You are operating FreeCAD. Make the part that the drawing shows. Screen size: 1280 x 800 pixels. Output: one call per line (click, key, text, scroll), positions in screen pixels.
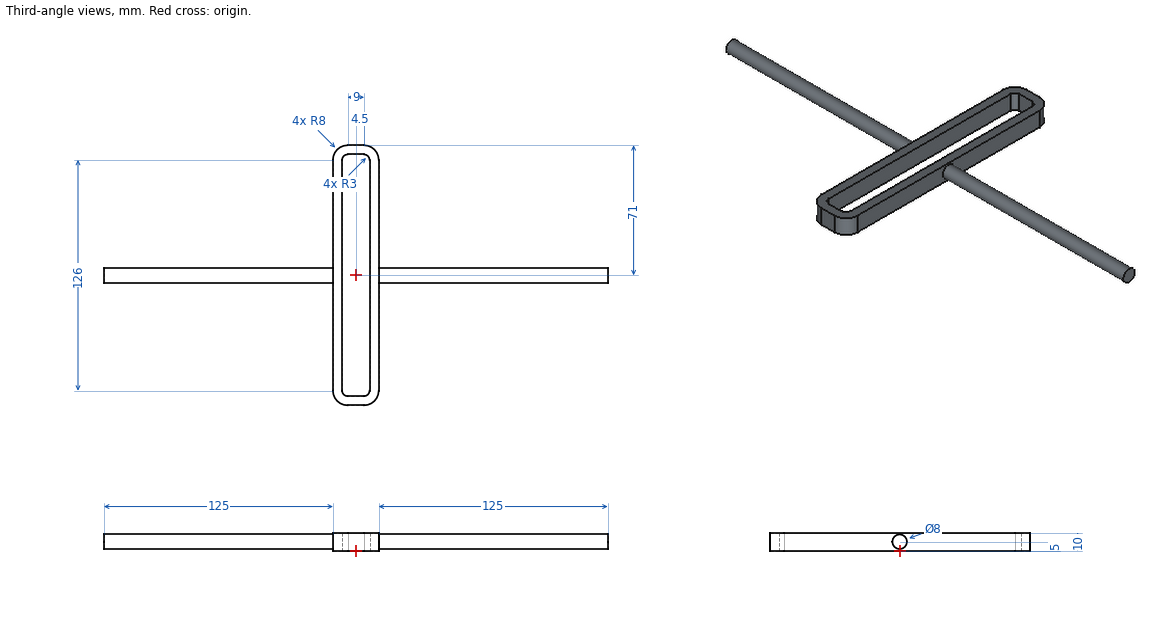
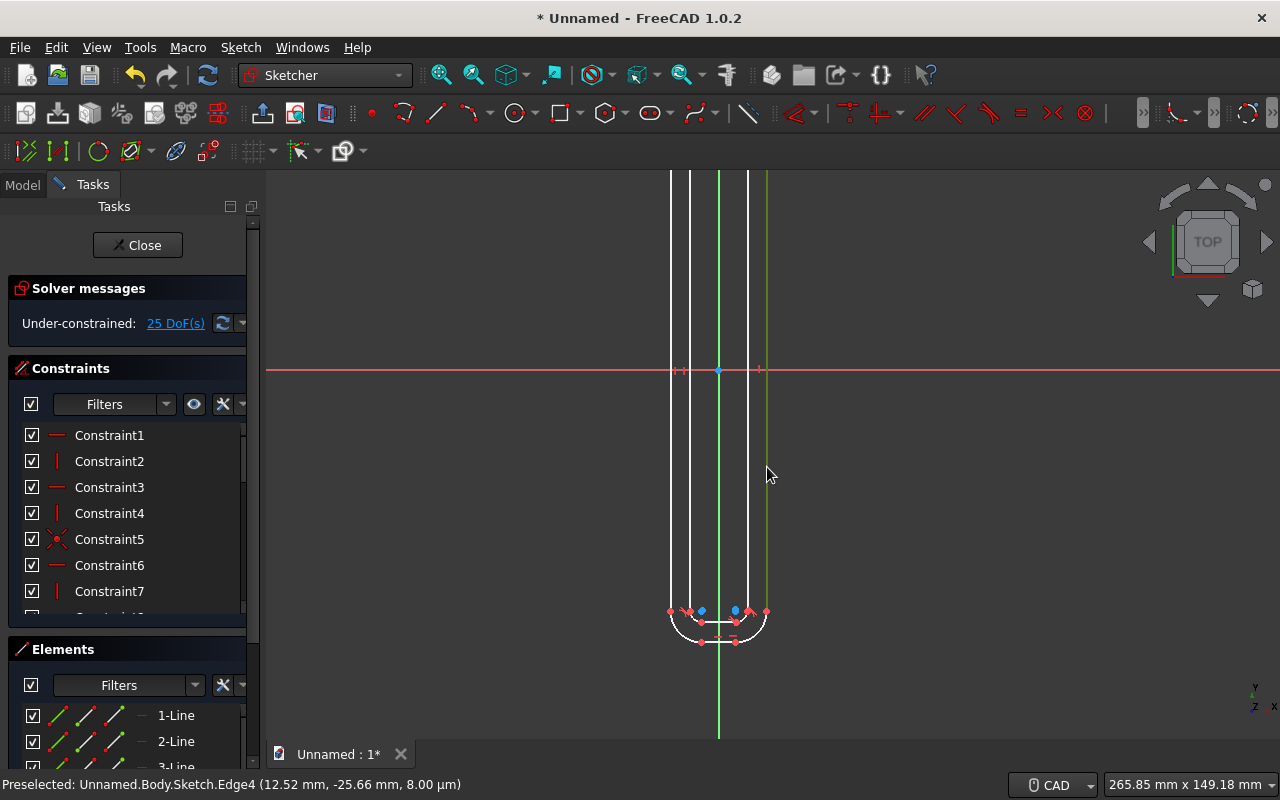
scroll(675, 626, down, 2)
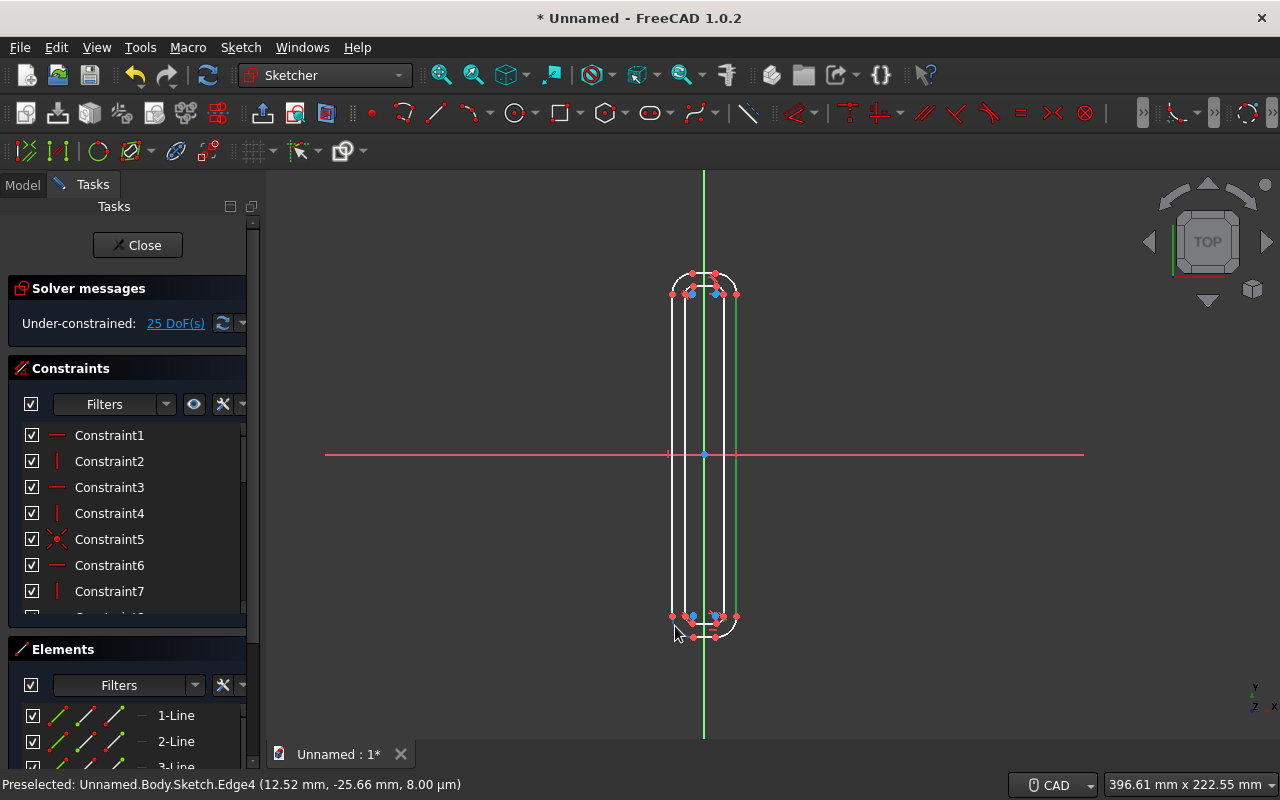
scroll(734, 285, up, 2)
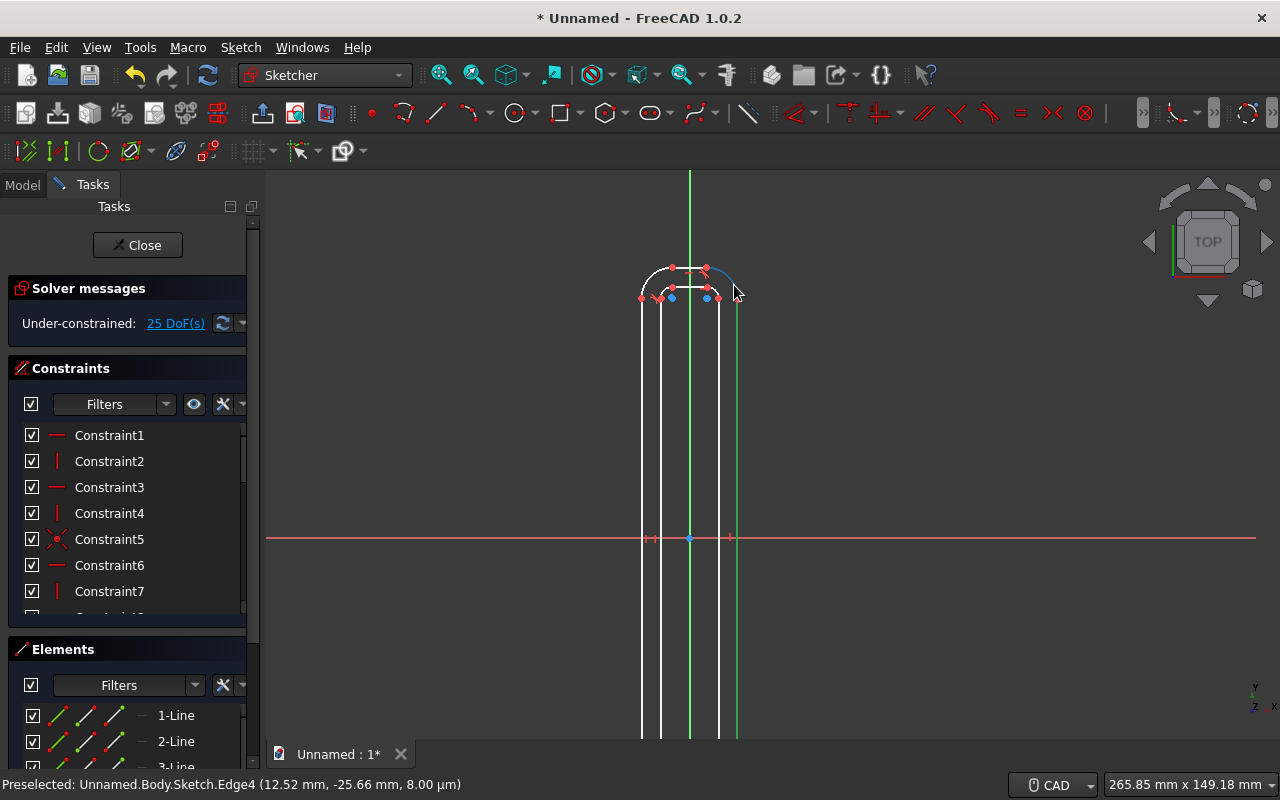
click(734, 285)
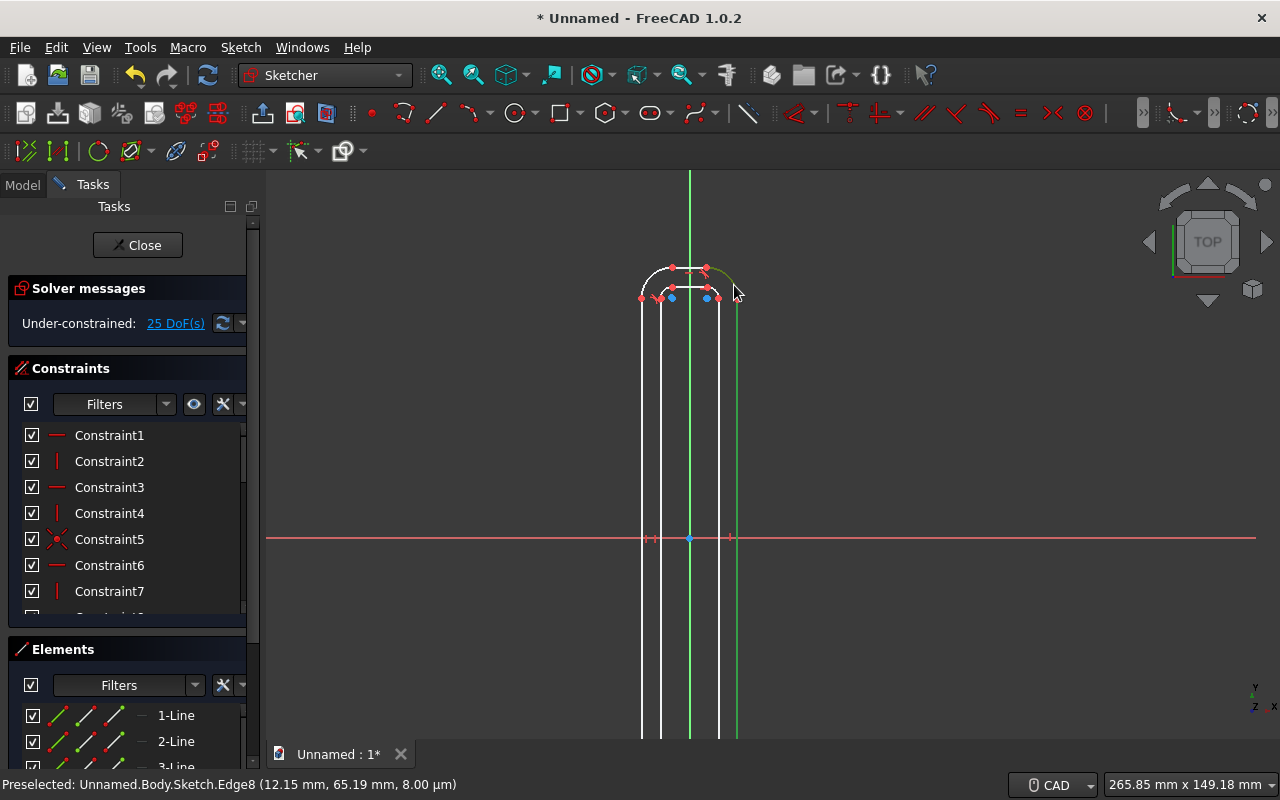
click(990, 114)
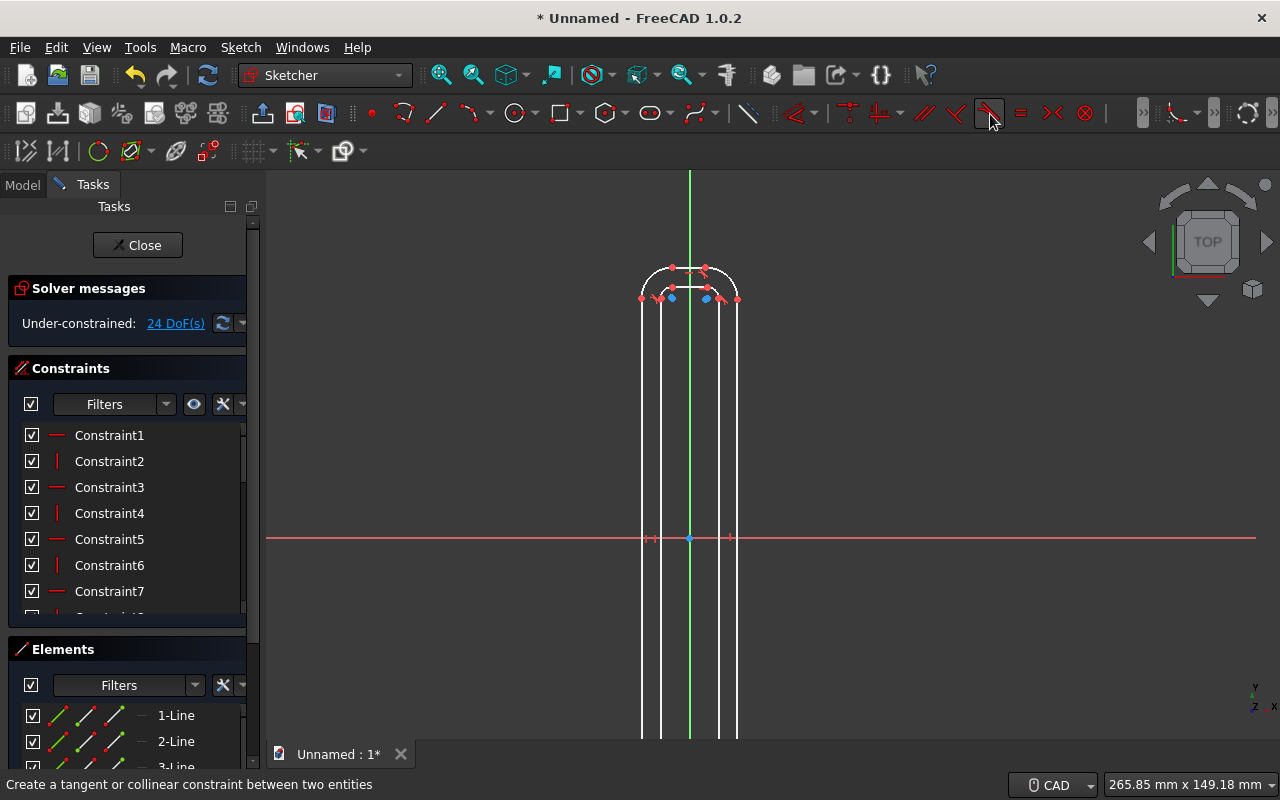
click(686, 287)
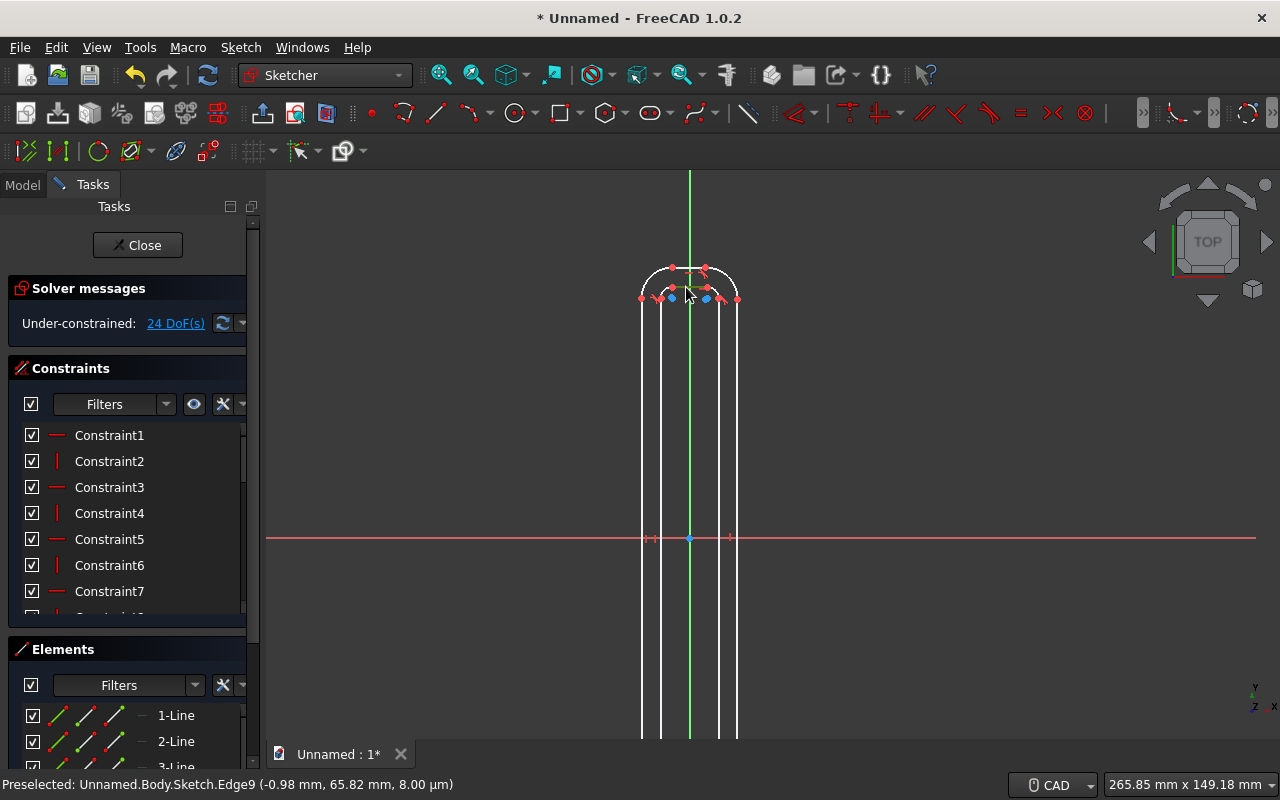
scroll(715, 290, up, 3)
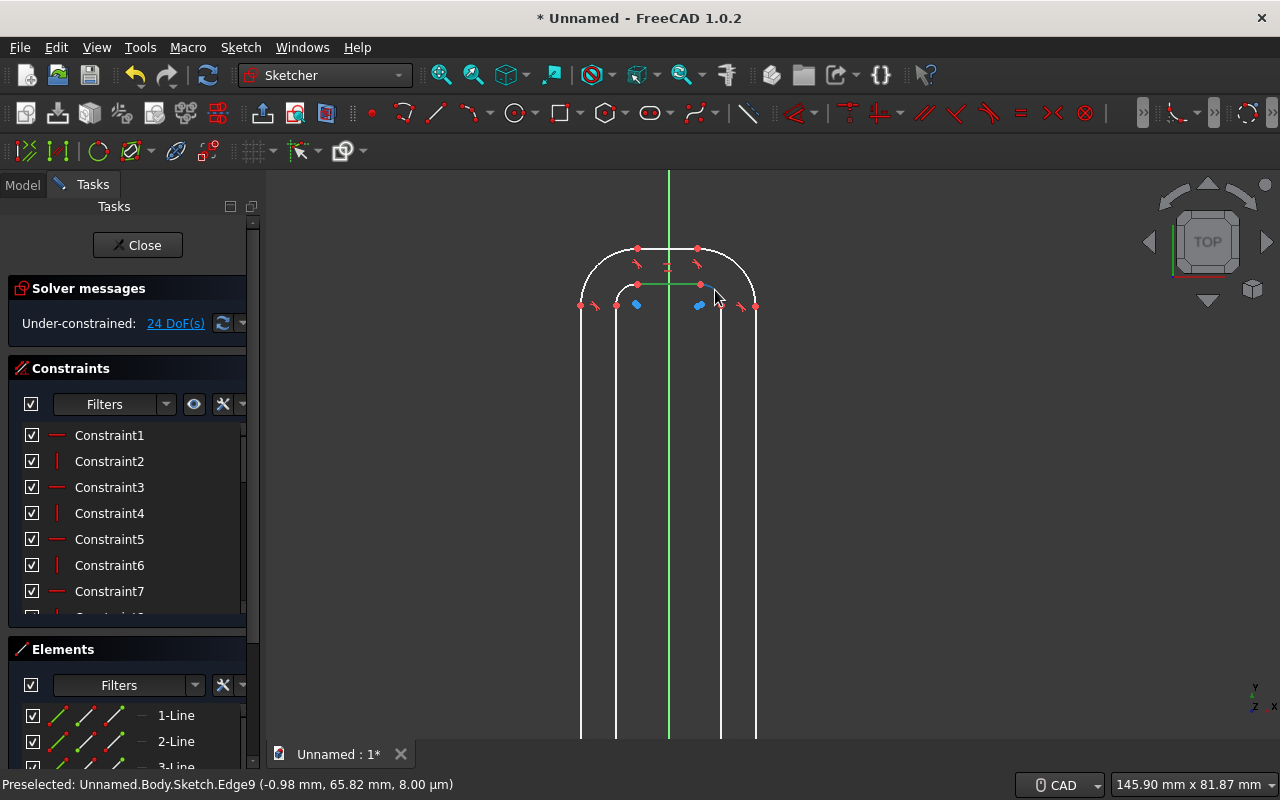
click(715, 290)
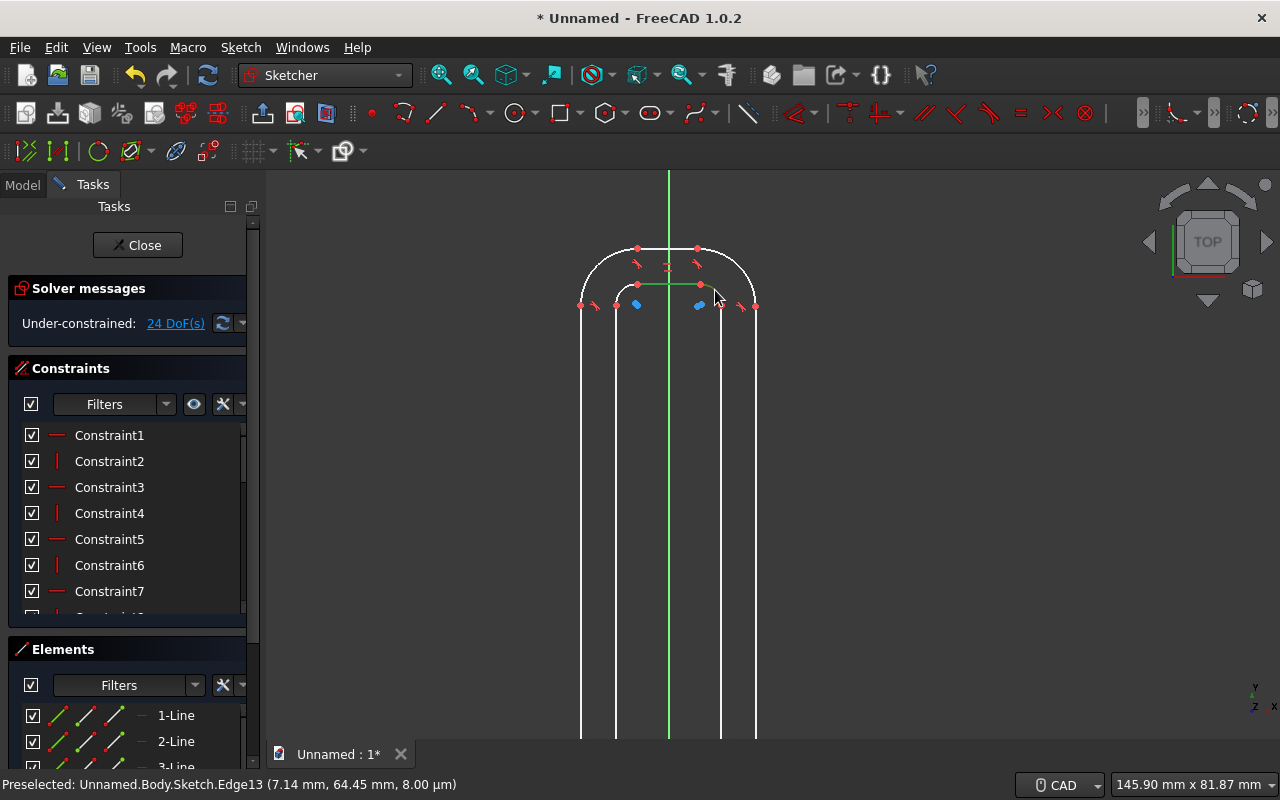
click(990, 114)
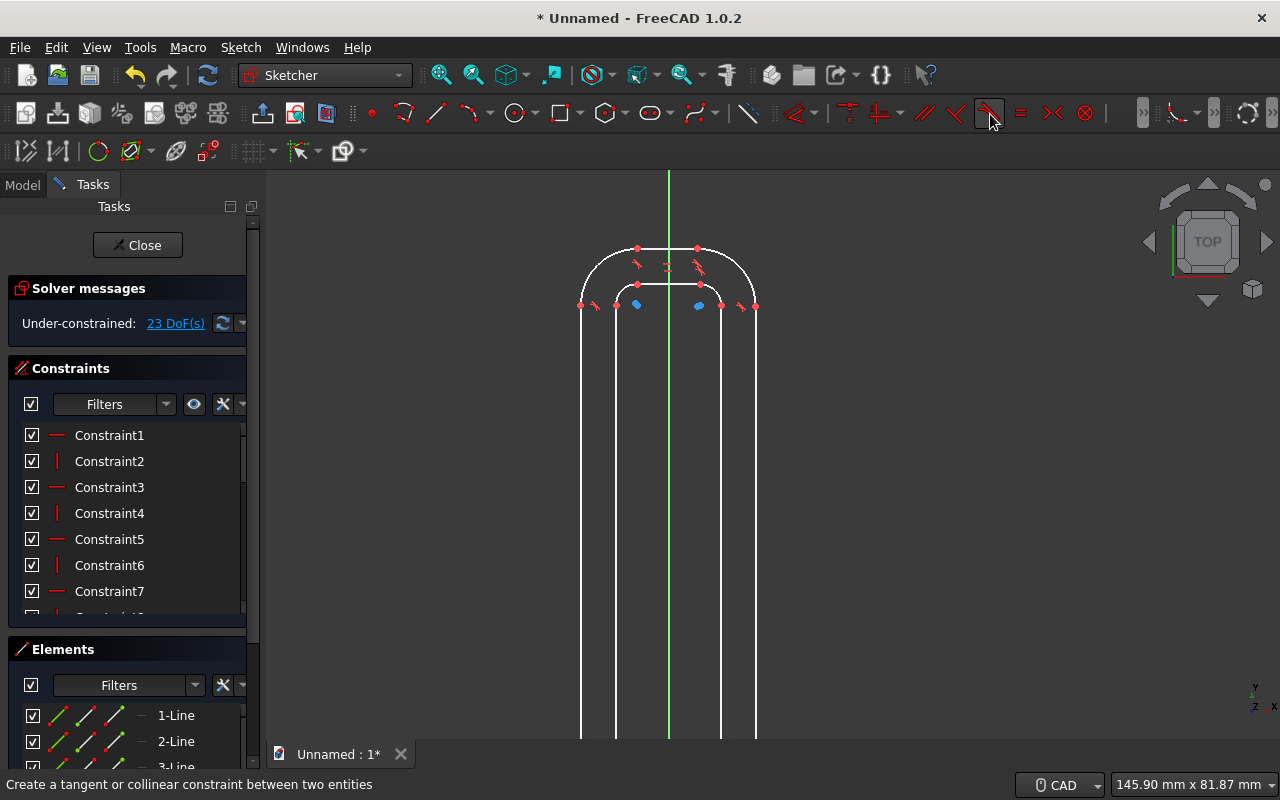
click(656, 284)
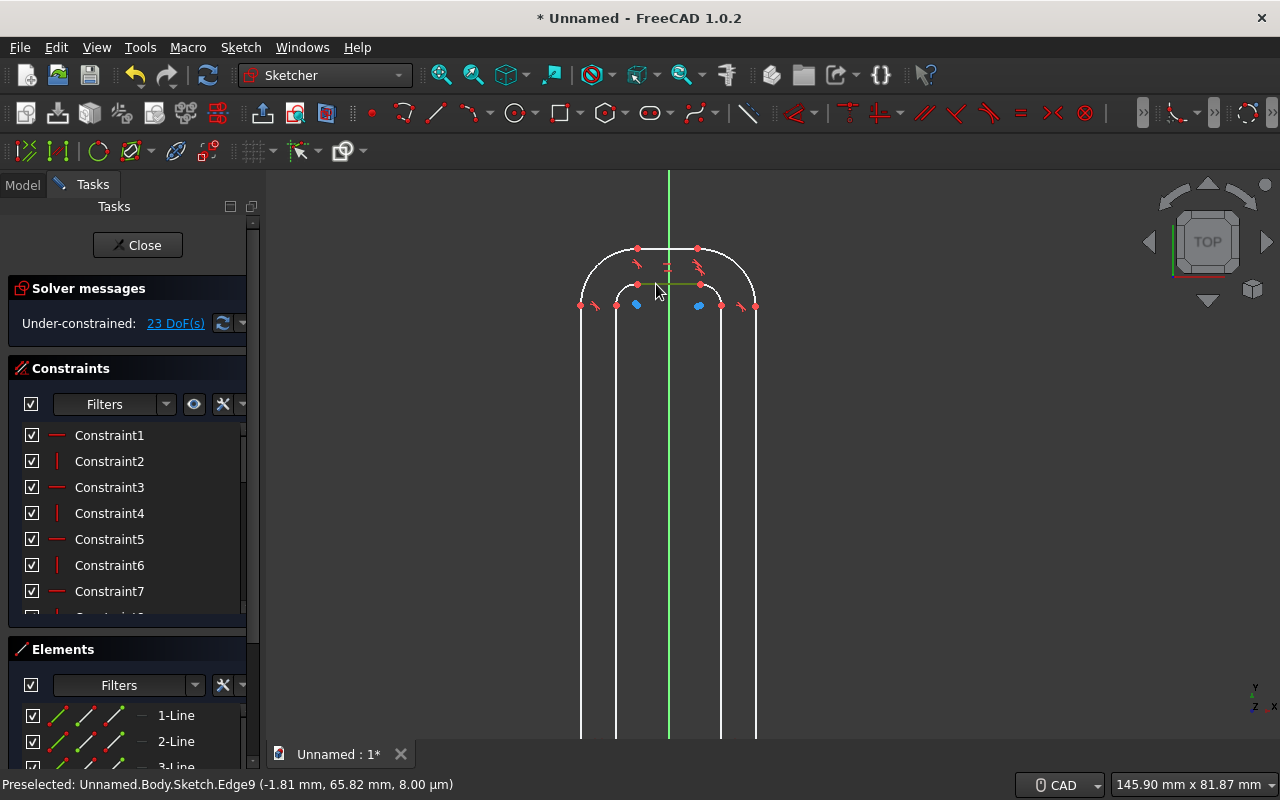
scroll(628, 286, up, 2)